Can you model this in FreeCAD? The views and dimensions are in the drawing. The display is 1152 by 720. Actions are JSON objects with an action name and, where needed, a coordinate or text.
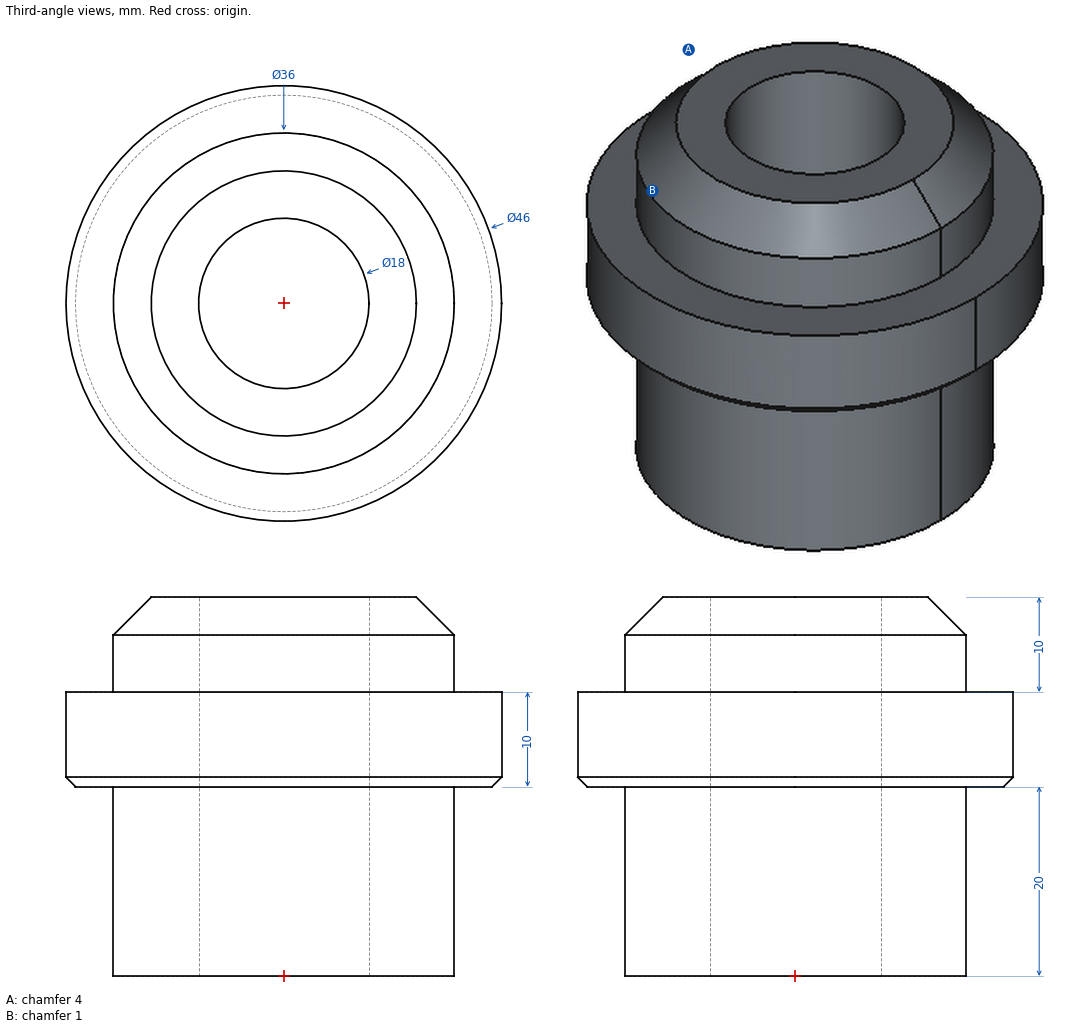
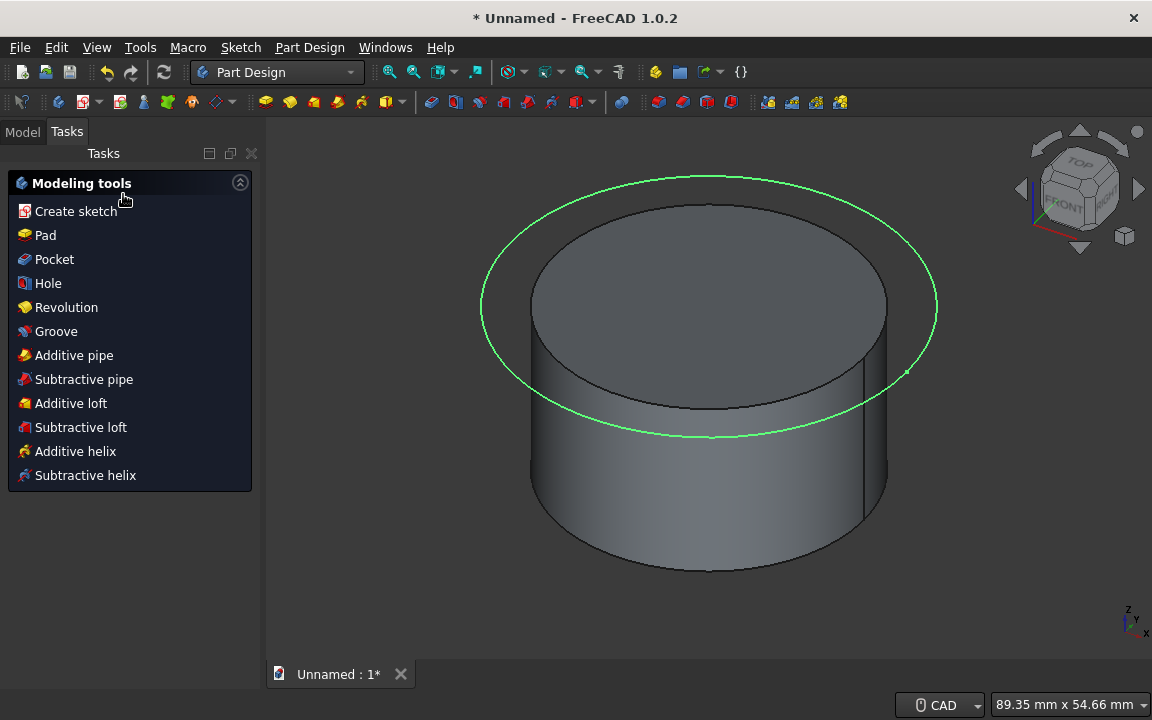
{"action": "left_click", "coordinate": [266, 102]}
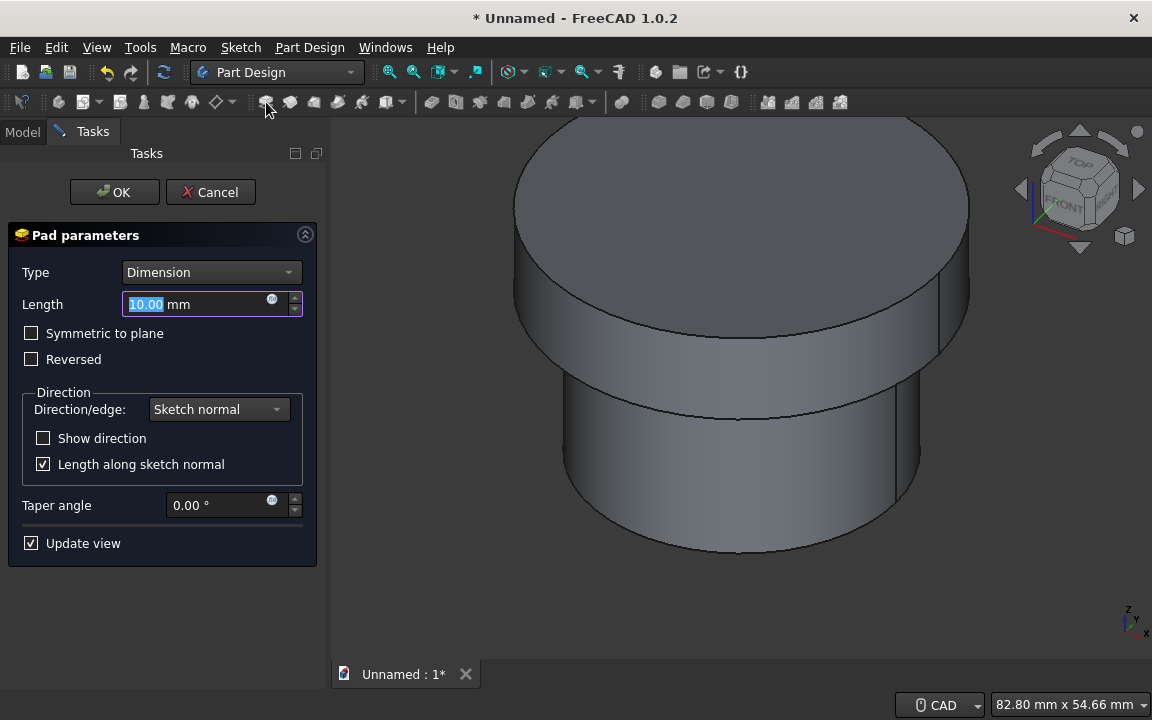
{"action": "type", "text": "10"}
{"action": "key", "text": "Tab"}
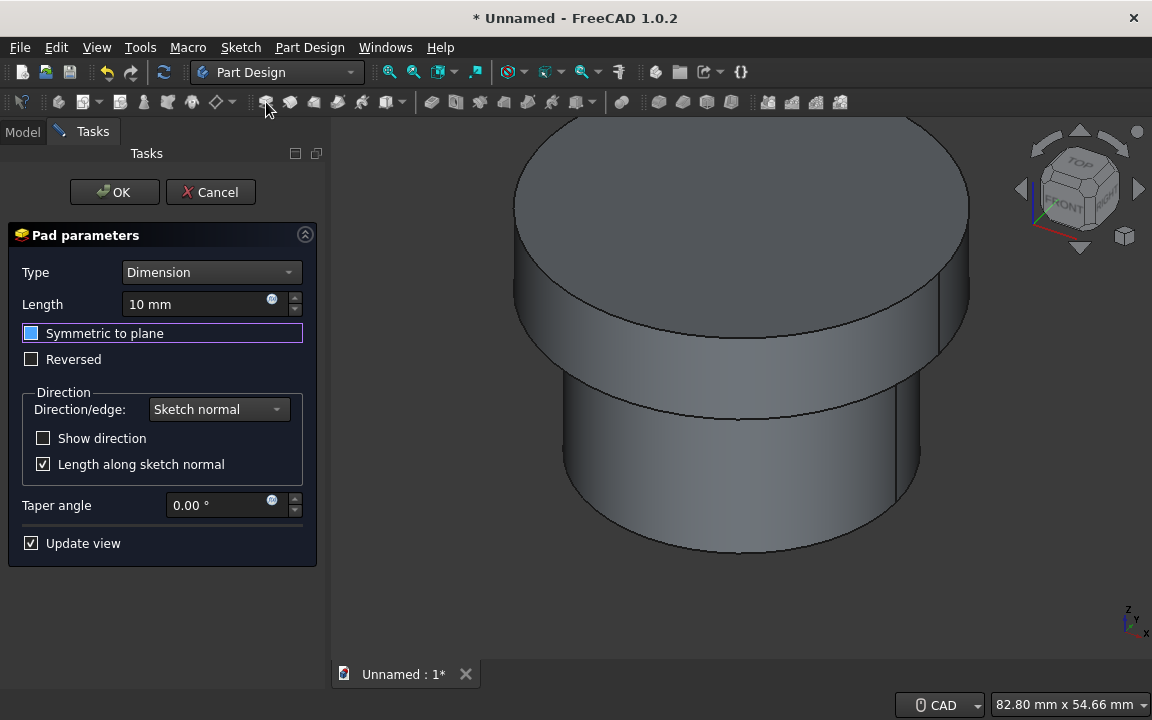
{"action": "left_click", "coordinate": [115, 192]}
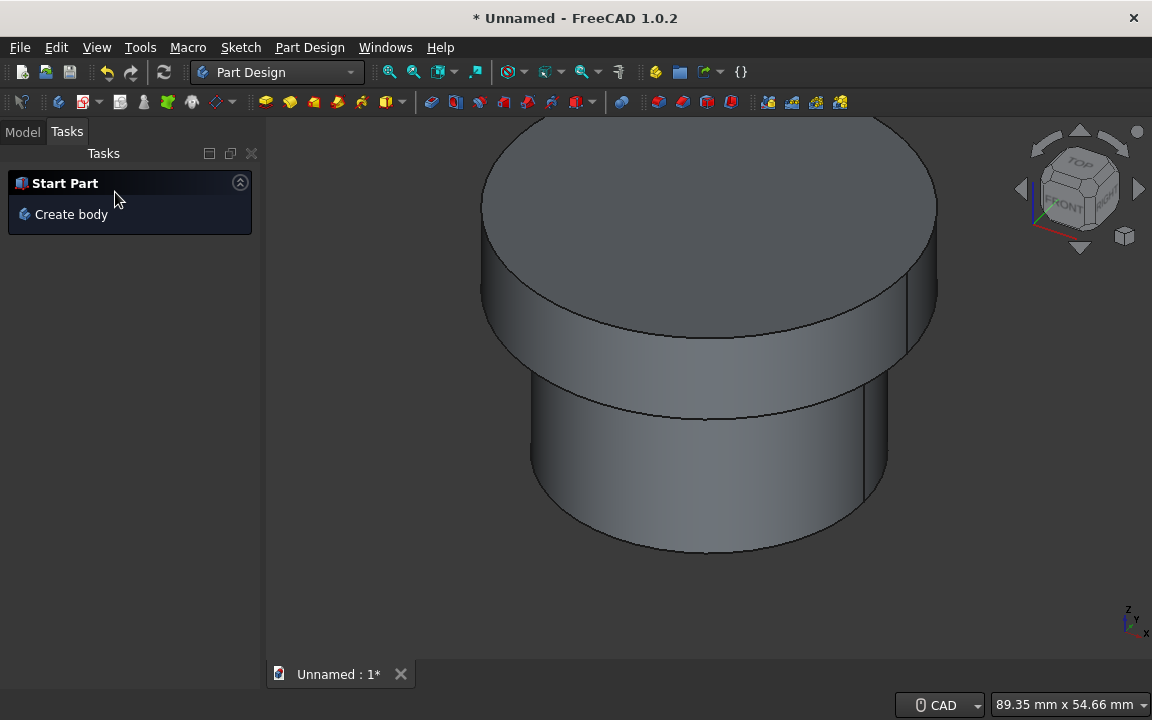
{"action": "key", "text": "v f"}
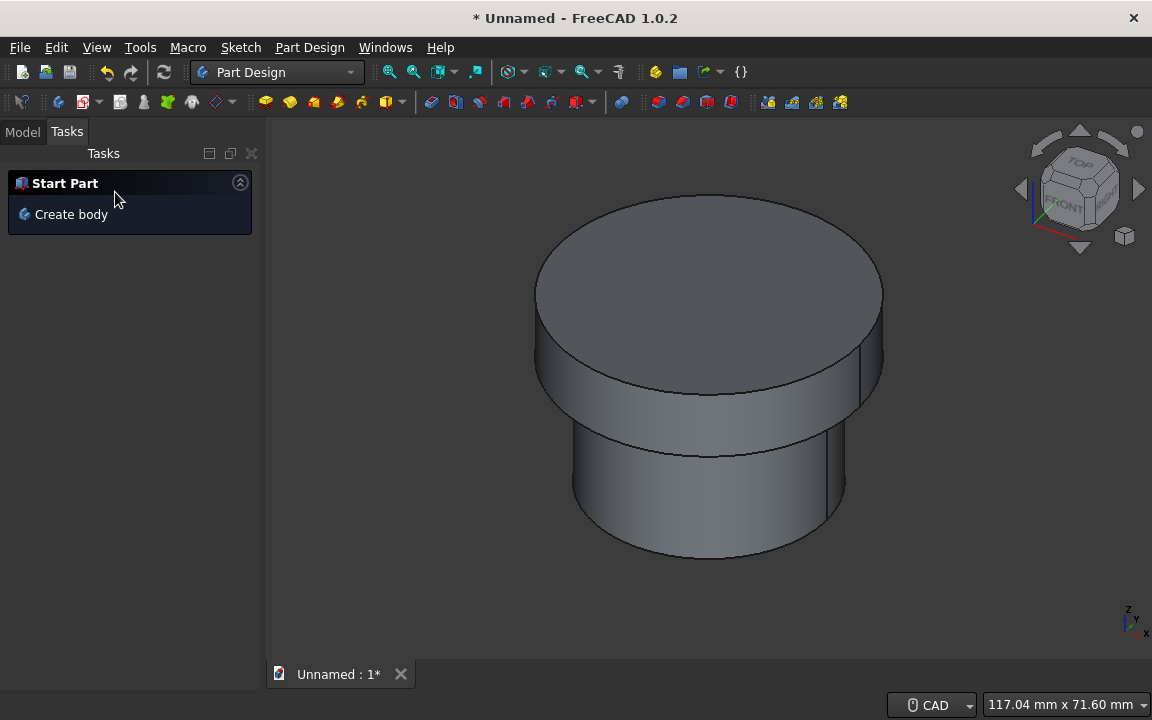
{"action": "left_click", "coordinate": [709, 294]}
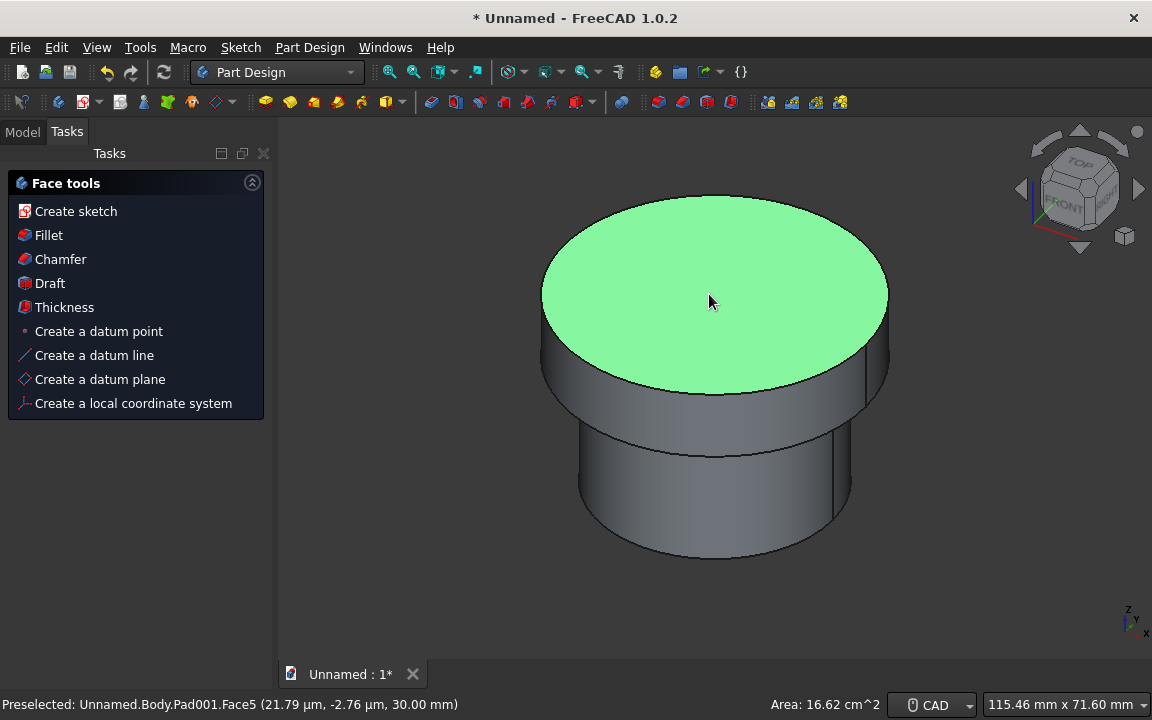
{"action": "left_click", "coordinate": [84, 102]}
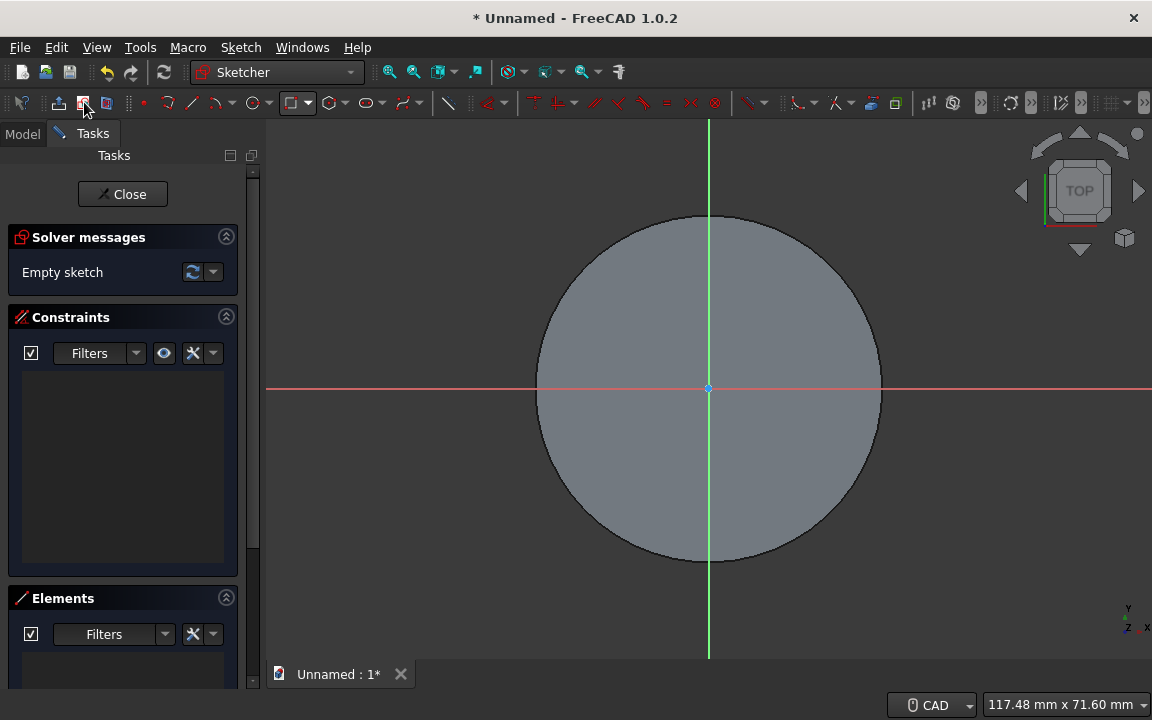
{"action": "left_click", "coordinate": [254, 104]}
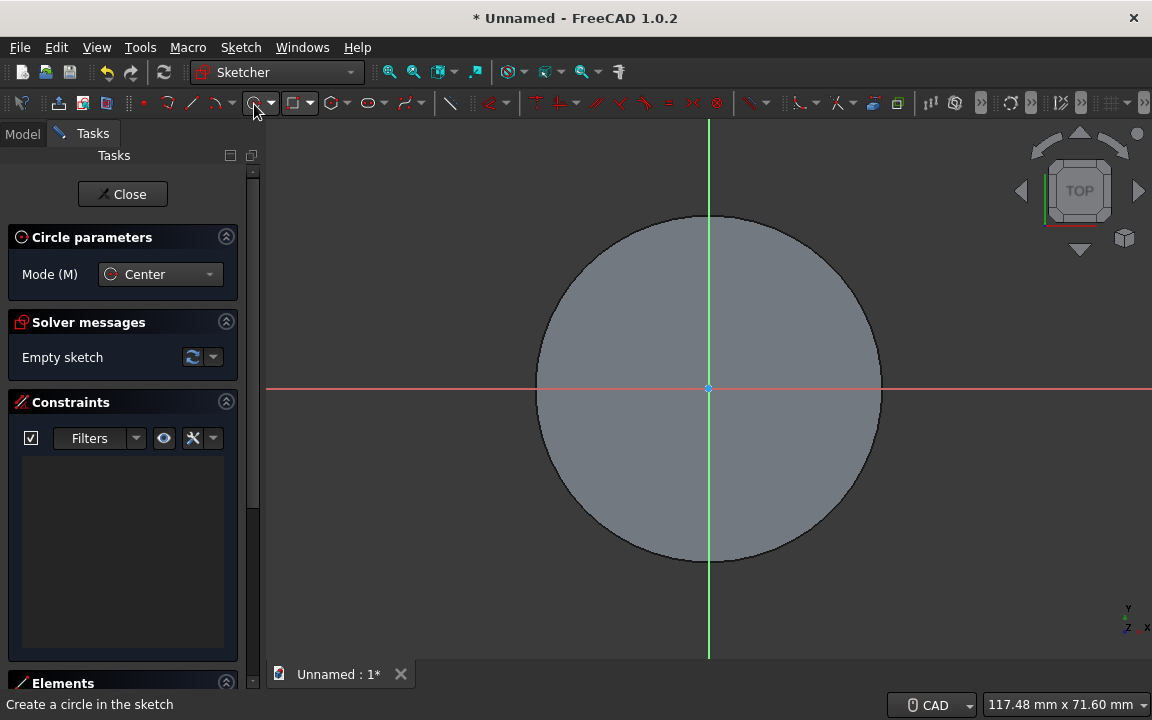
{"action": "left_click", "coordinate": [709, 389]}
{"action": "left_click", "coordinate": [805, 293]}
{"action": "key", "text": "Escape"}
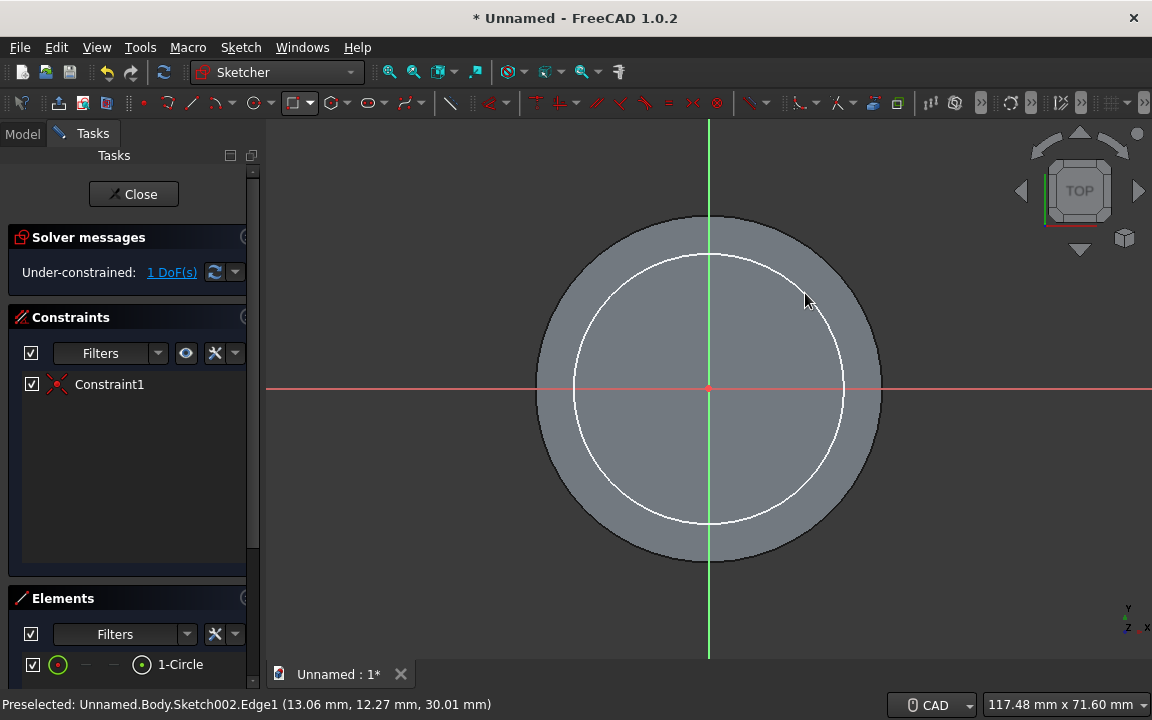
{"action": "key", "text": "d"}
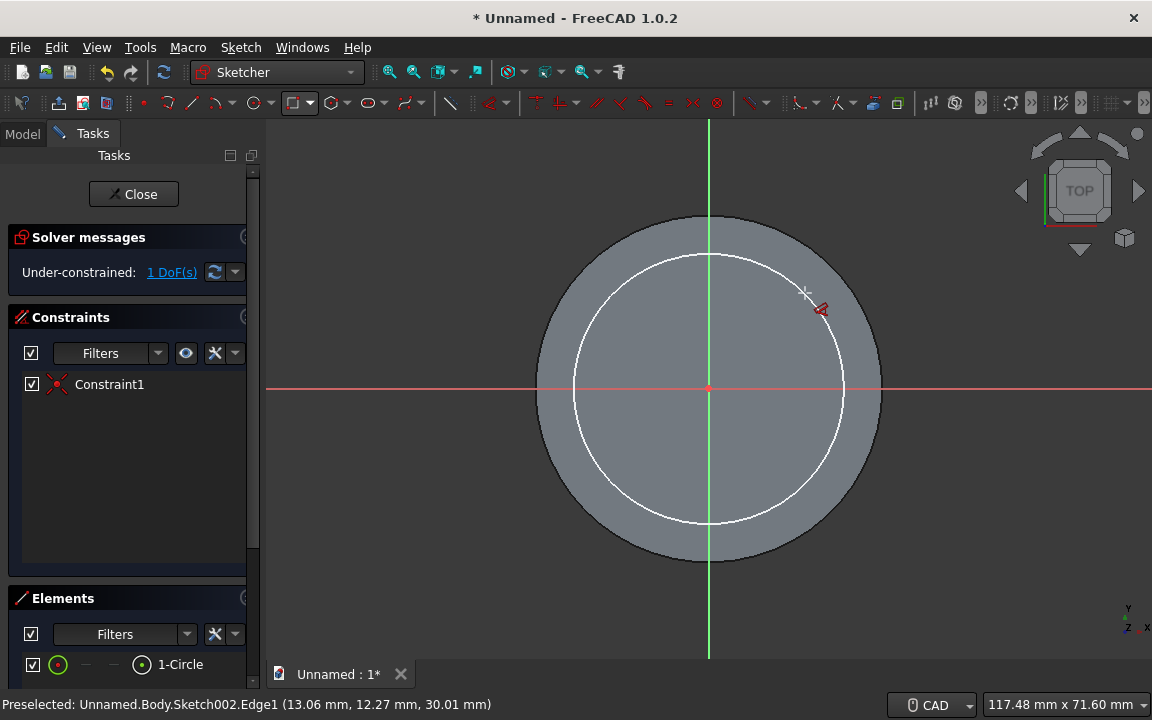
{"action": "left_click", "coordinate": [804, 293]}
{"action": "left_click", "coordinate": [827, 270]}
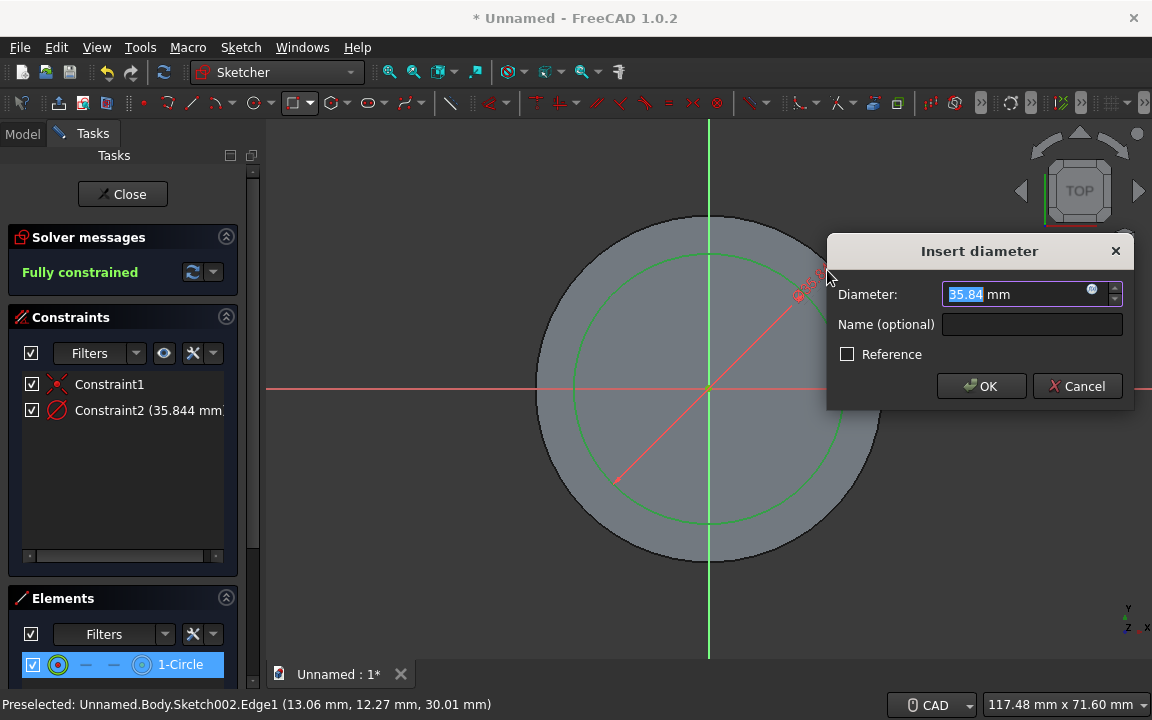
{"action": "type", "text": "36"}
{"action": "key", "text": "Return"}
{"action": "key", "text": "Escape"}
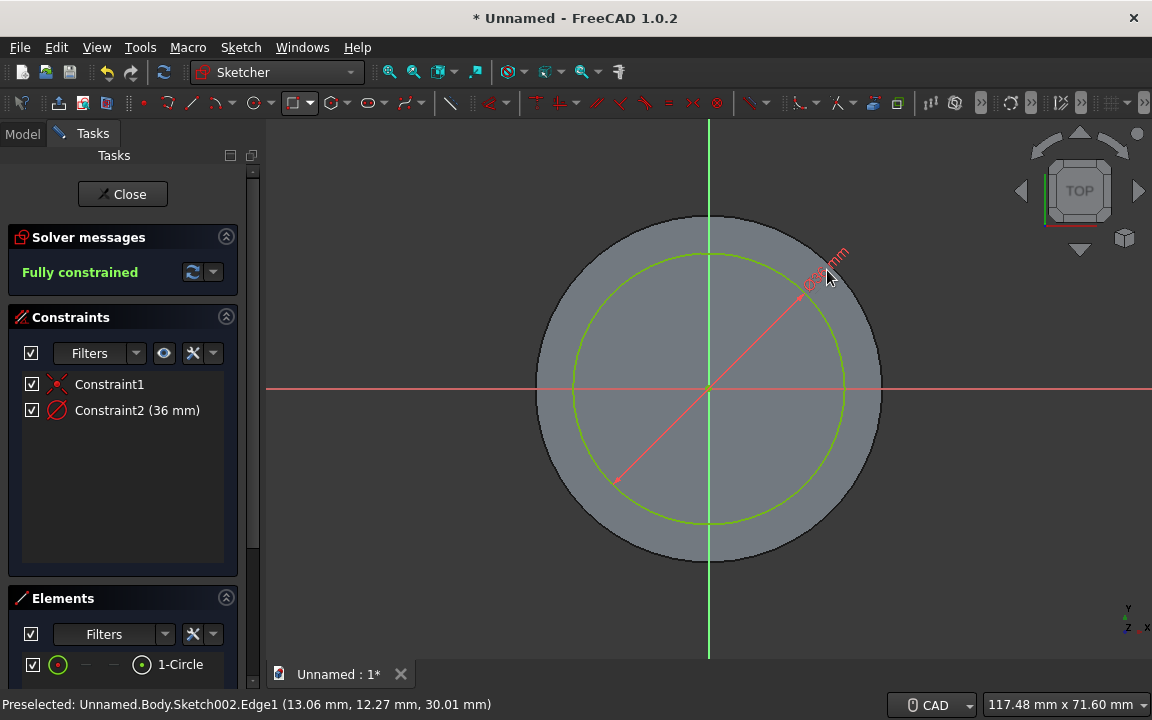
{"action": "left_click", "coordinate": [123, 194]}